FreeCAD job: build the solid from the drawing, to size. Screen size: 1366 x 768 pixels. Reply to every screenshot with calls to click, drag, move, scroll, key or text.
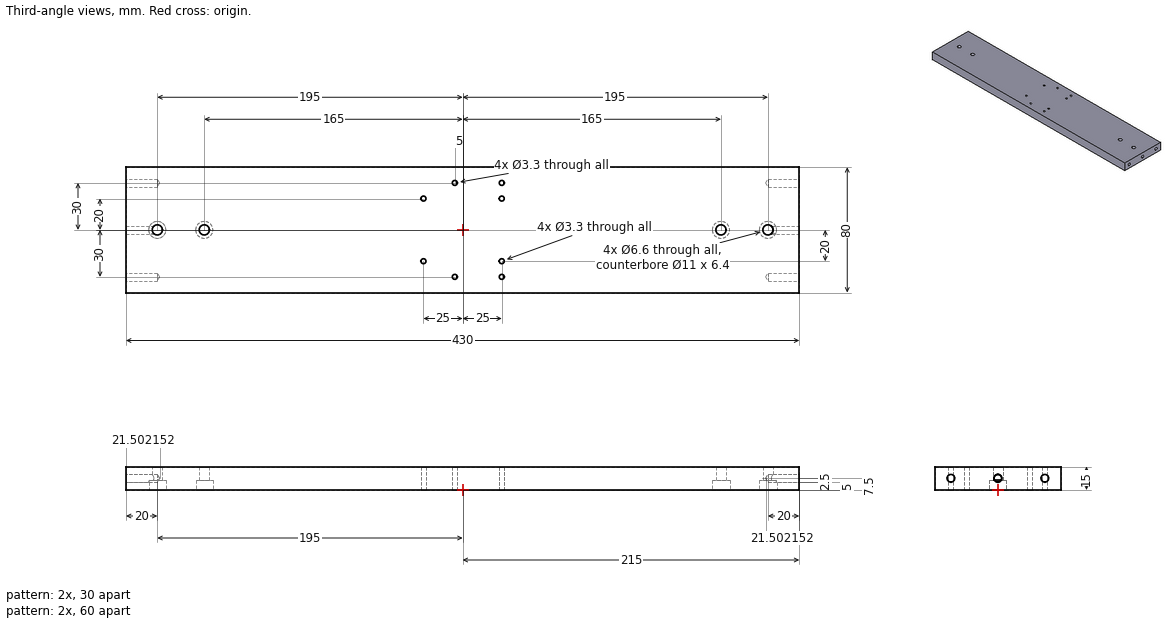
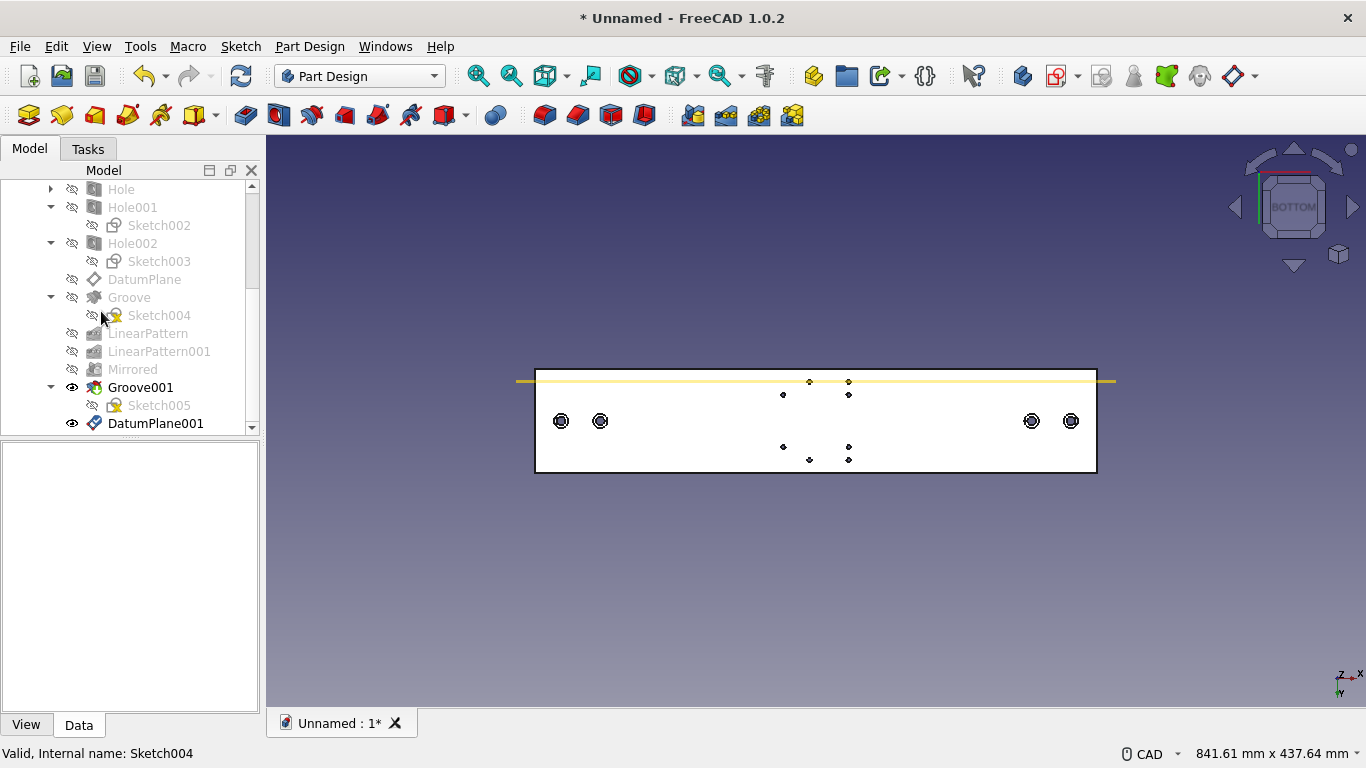
click(117, 423)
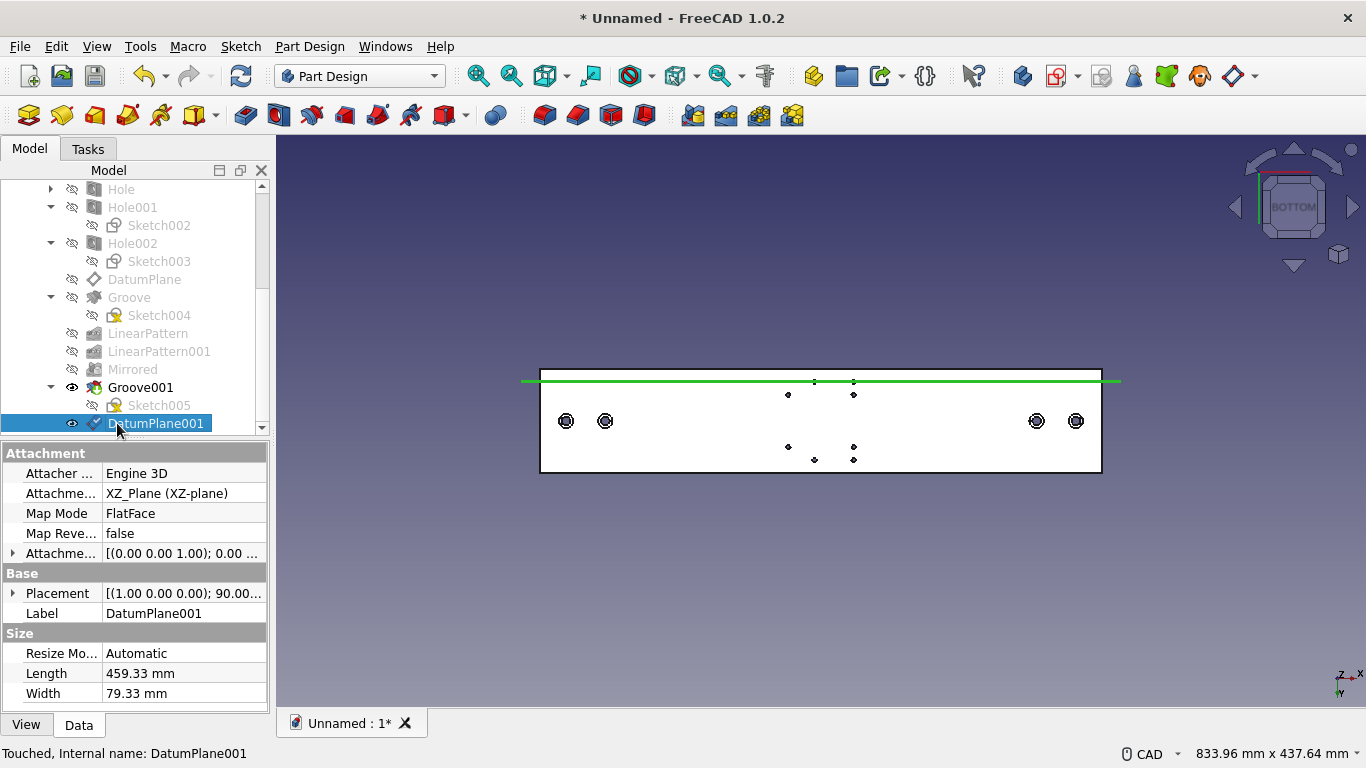
click(1056, 76)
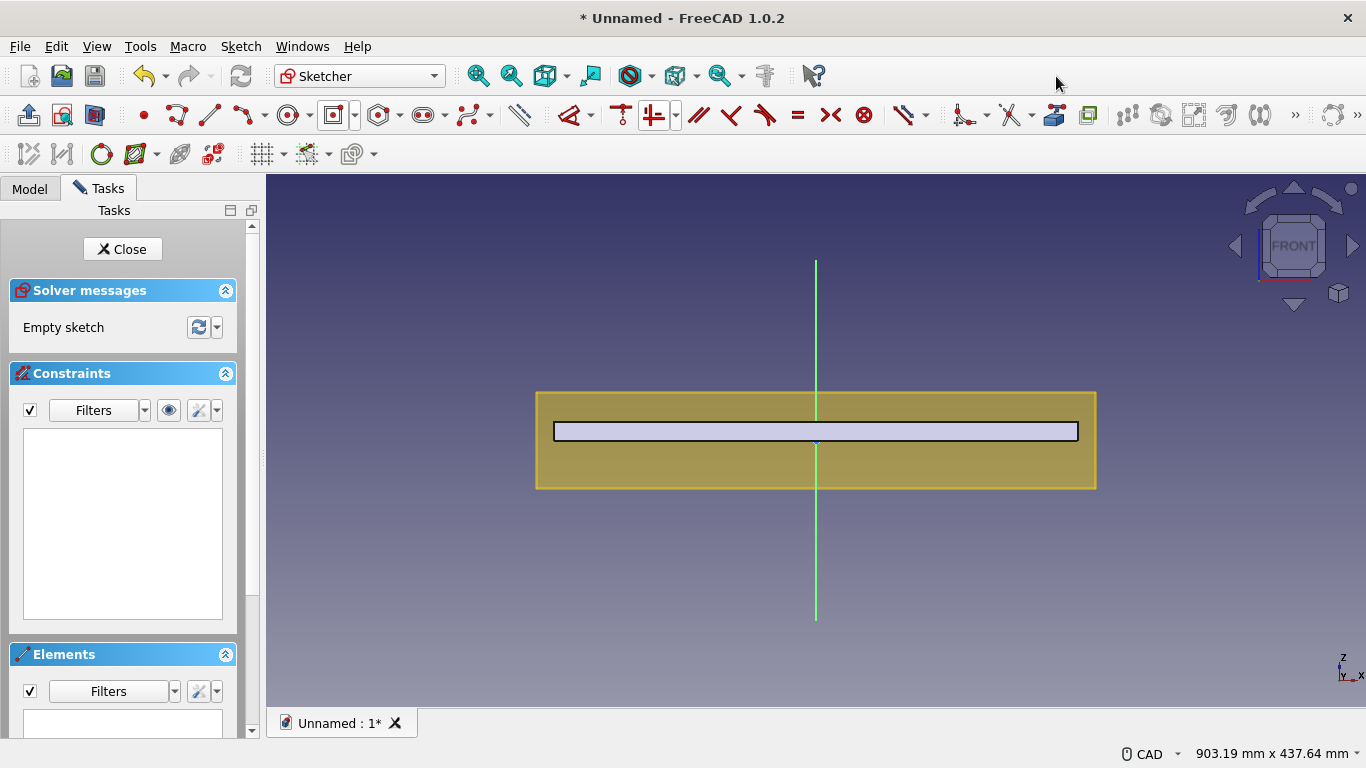
key(q)
key(s)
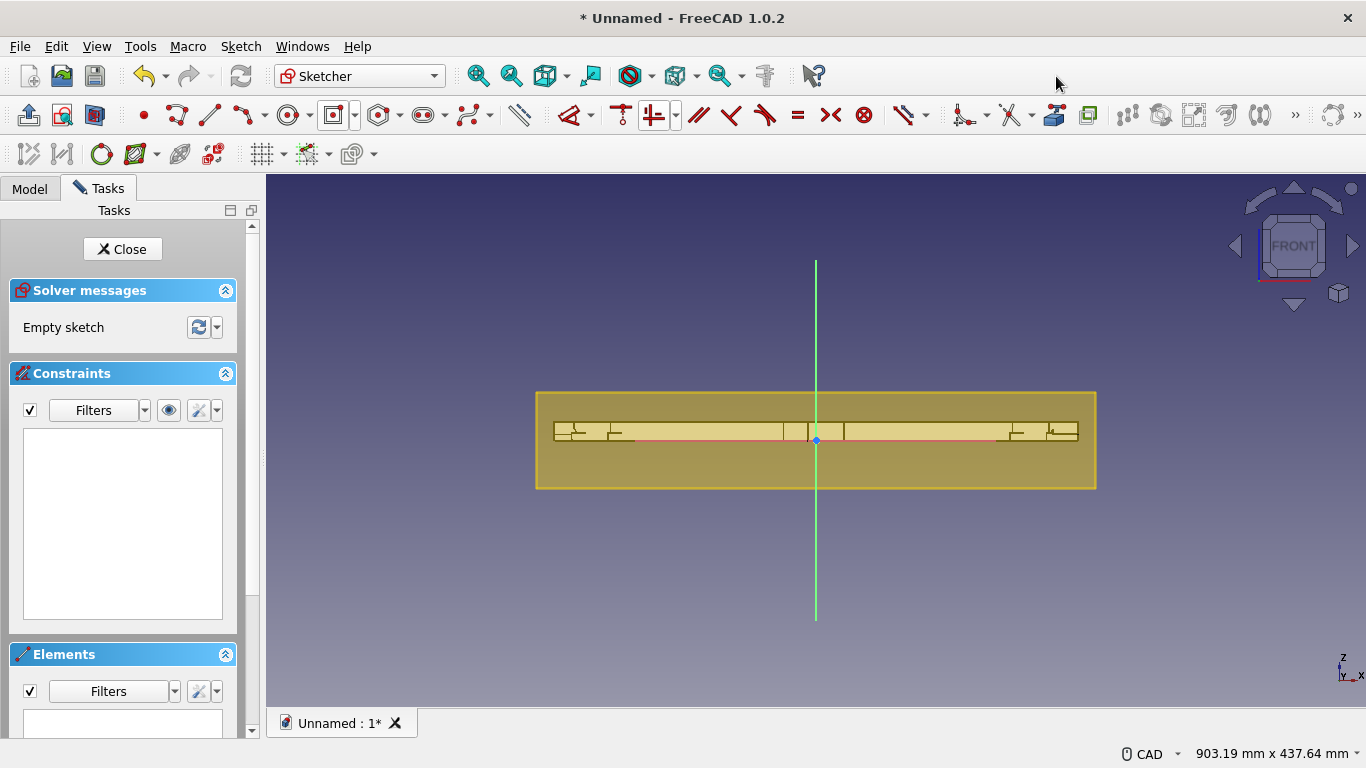
scroll(550, 432, up, 14)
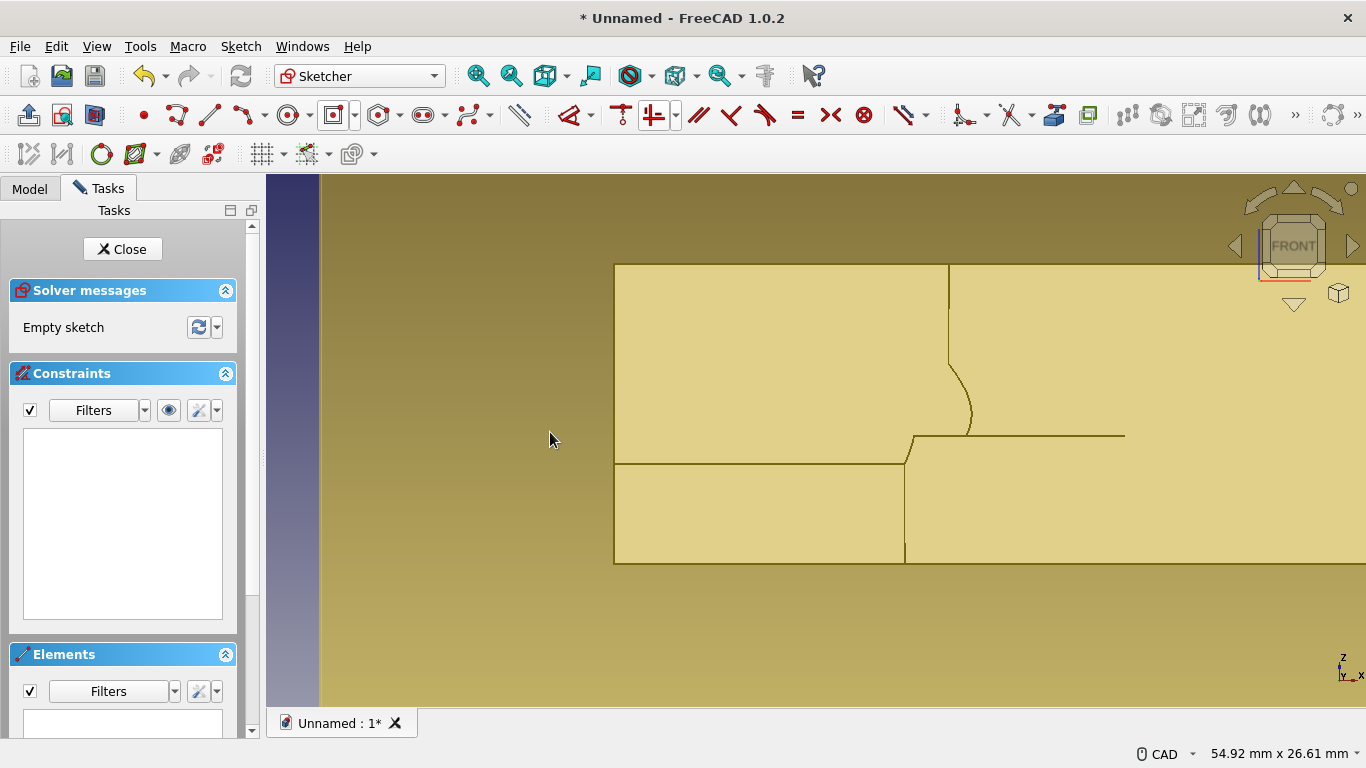
click(177, 116)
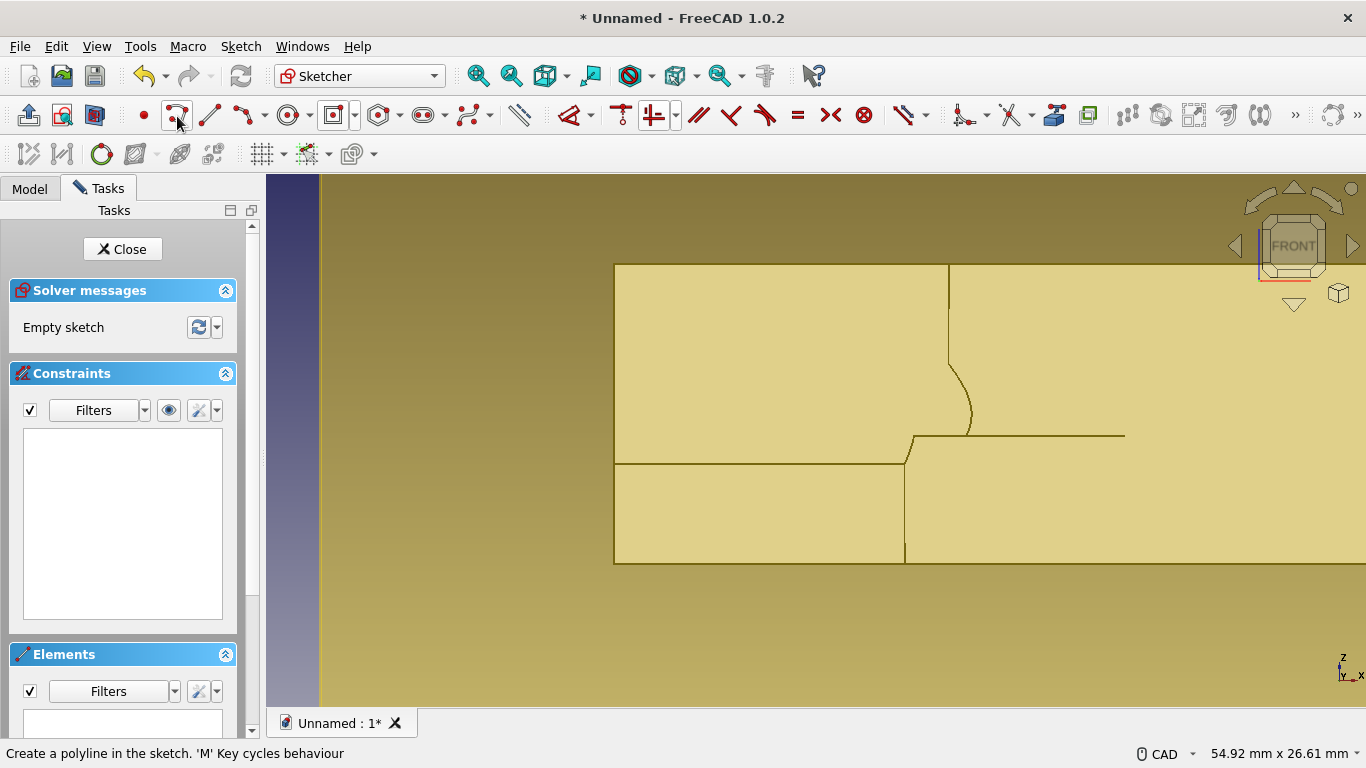
click(1045, 414)
click(1015, 464)
click(614, 464)
click(614, 414)
click(1045, 415)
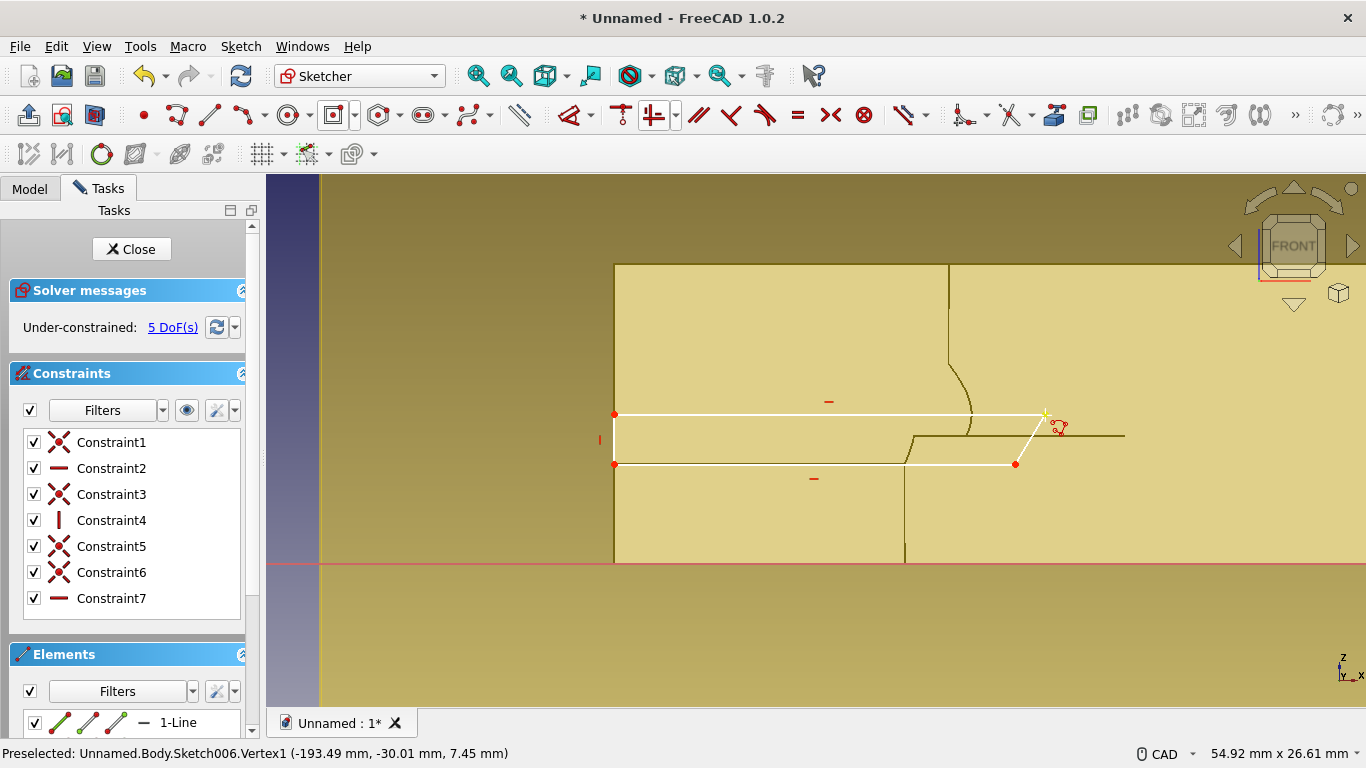
key(g)
key(l)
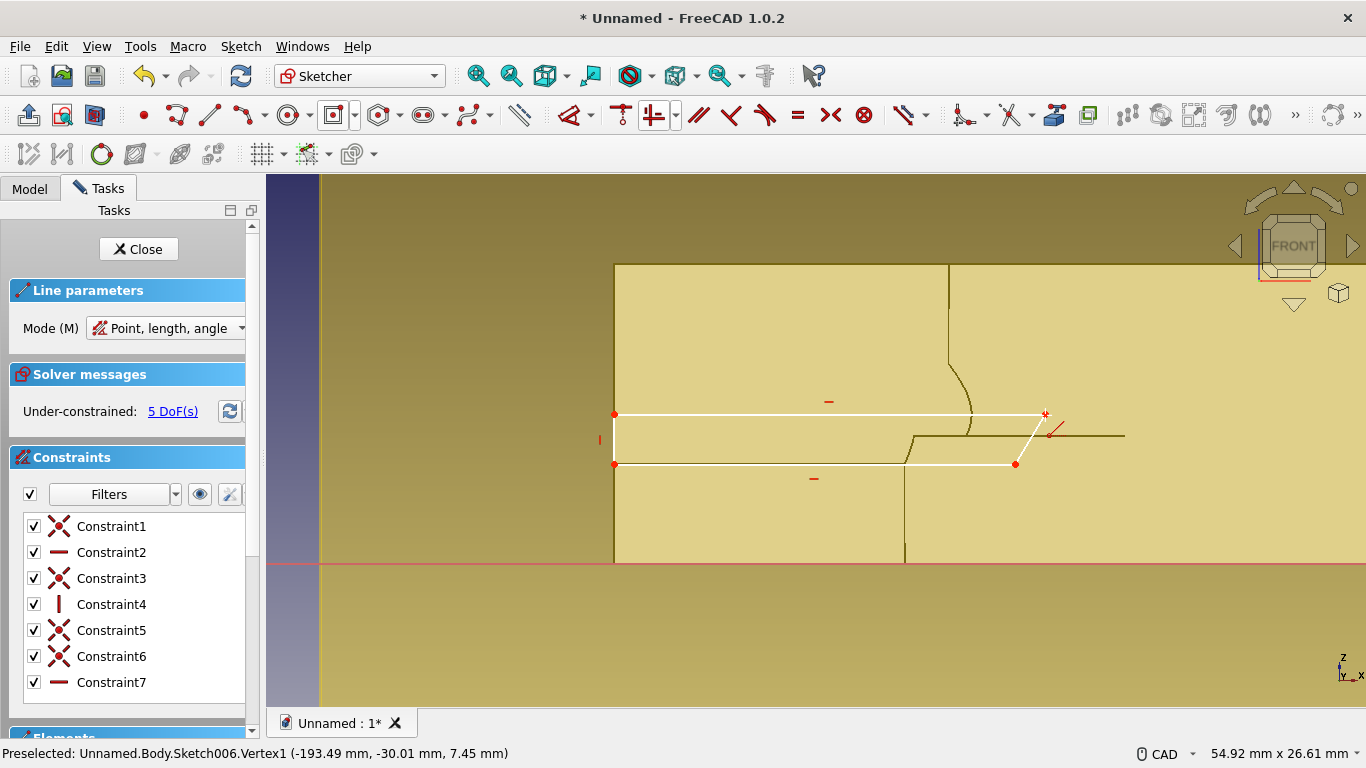
click(571, 414)
click(442, 414)
key(Escape)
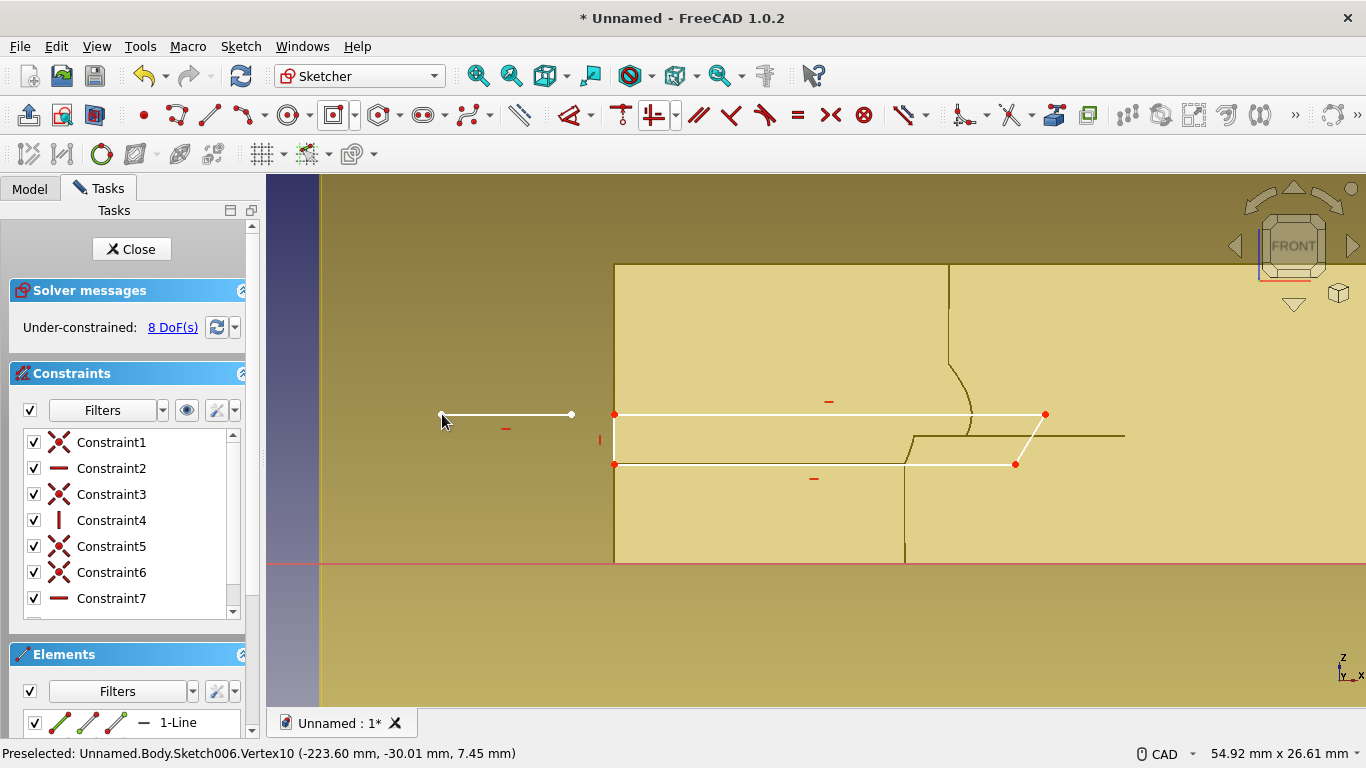
click(532, 415)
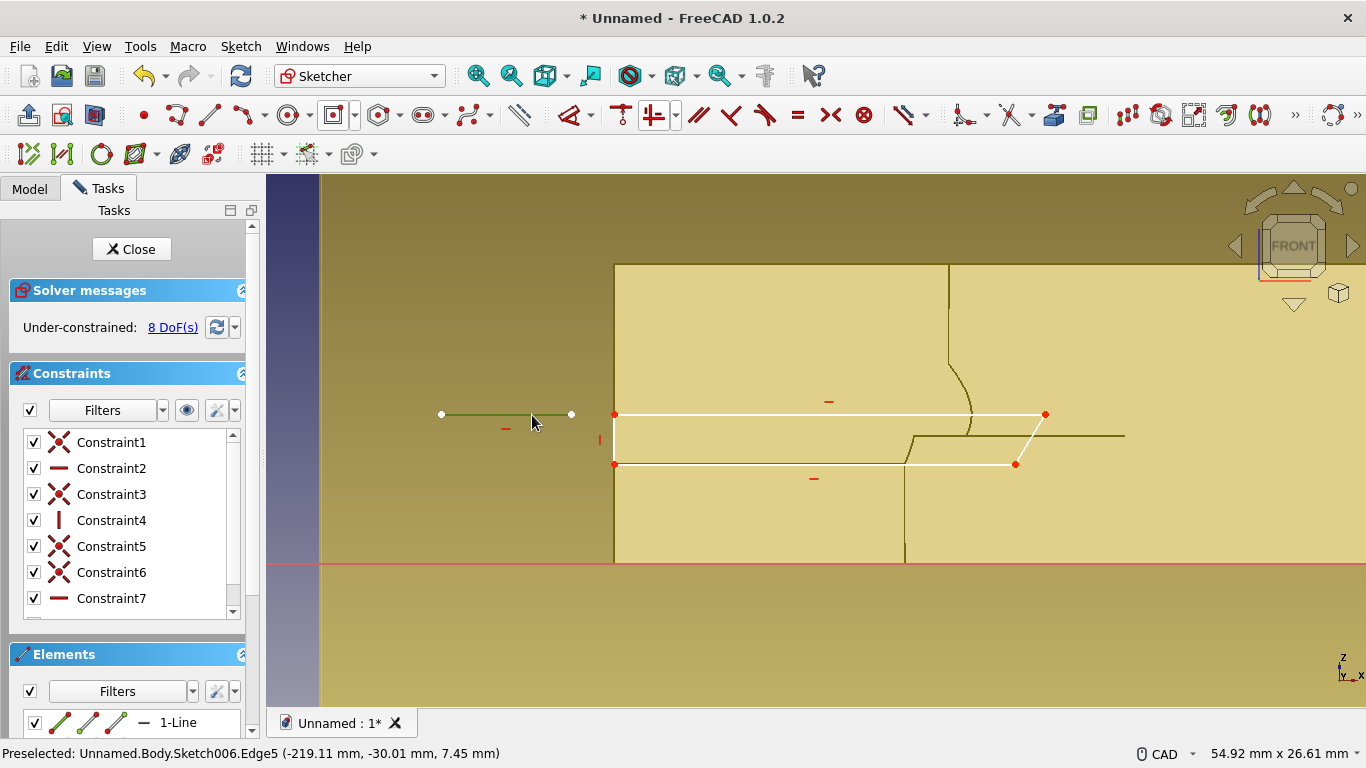
click(520, 116)